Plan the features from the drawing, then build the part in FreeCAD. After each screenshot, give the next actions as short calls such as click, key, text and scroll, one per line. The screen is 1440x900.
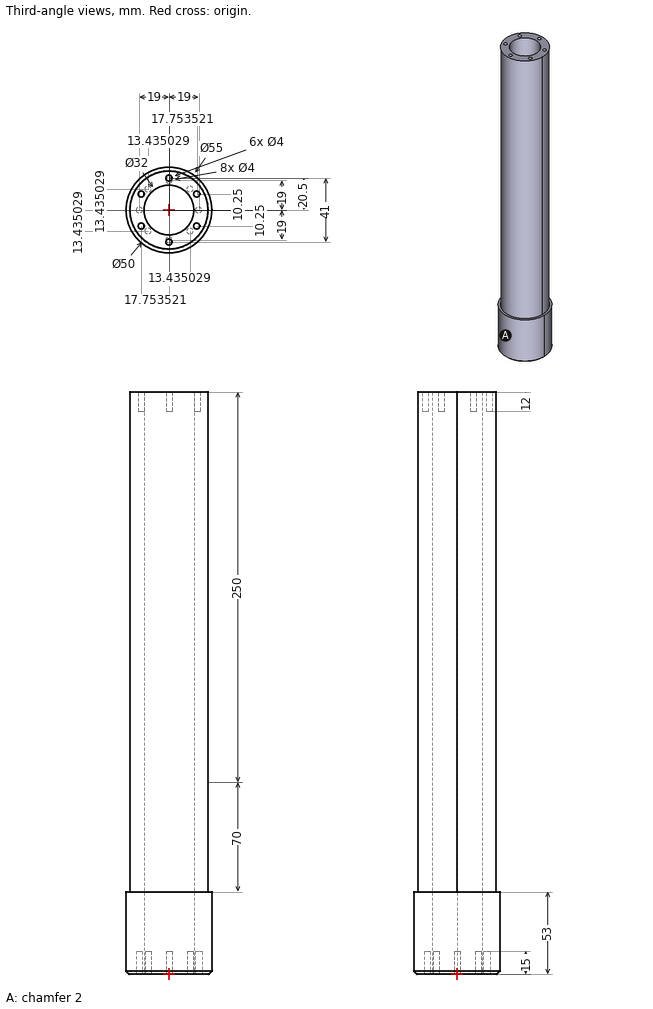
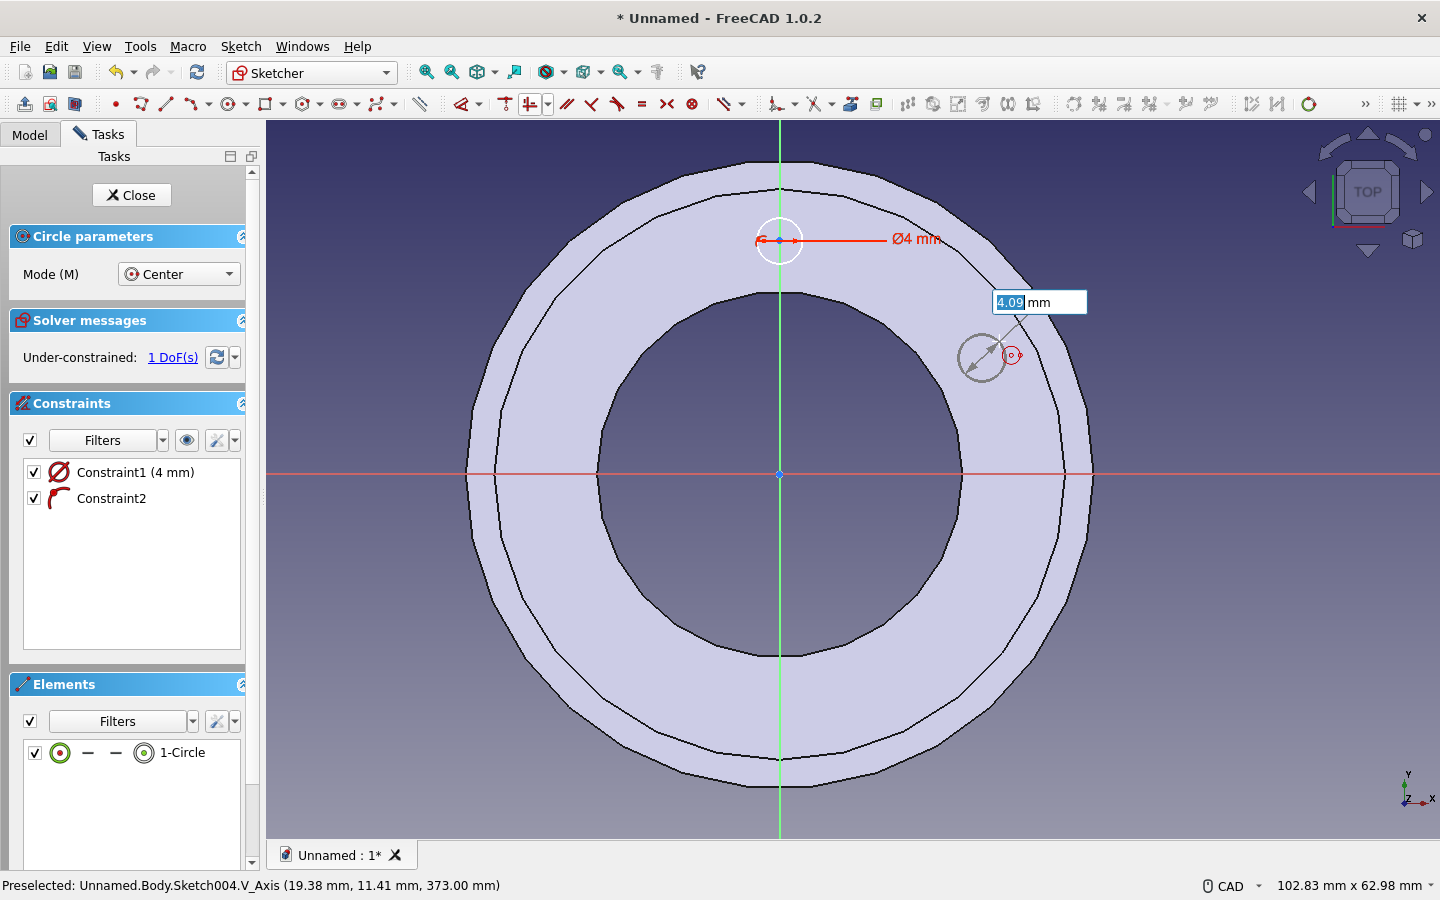
text(4)
key(Return)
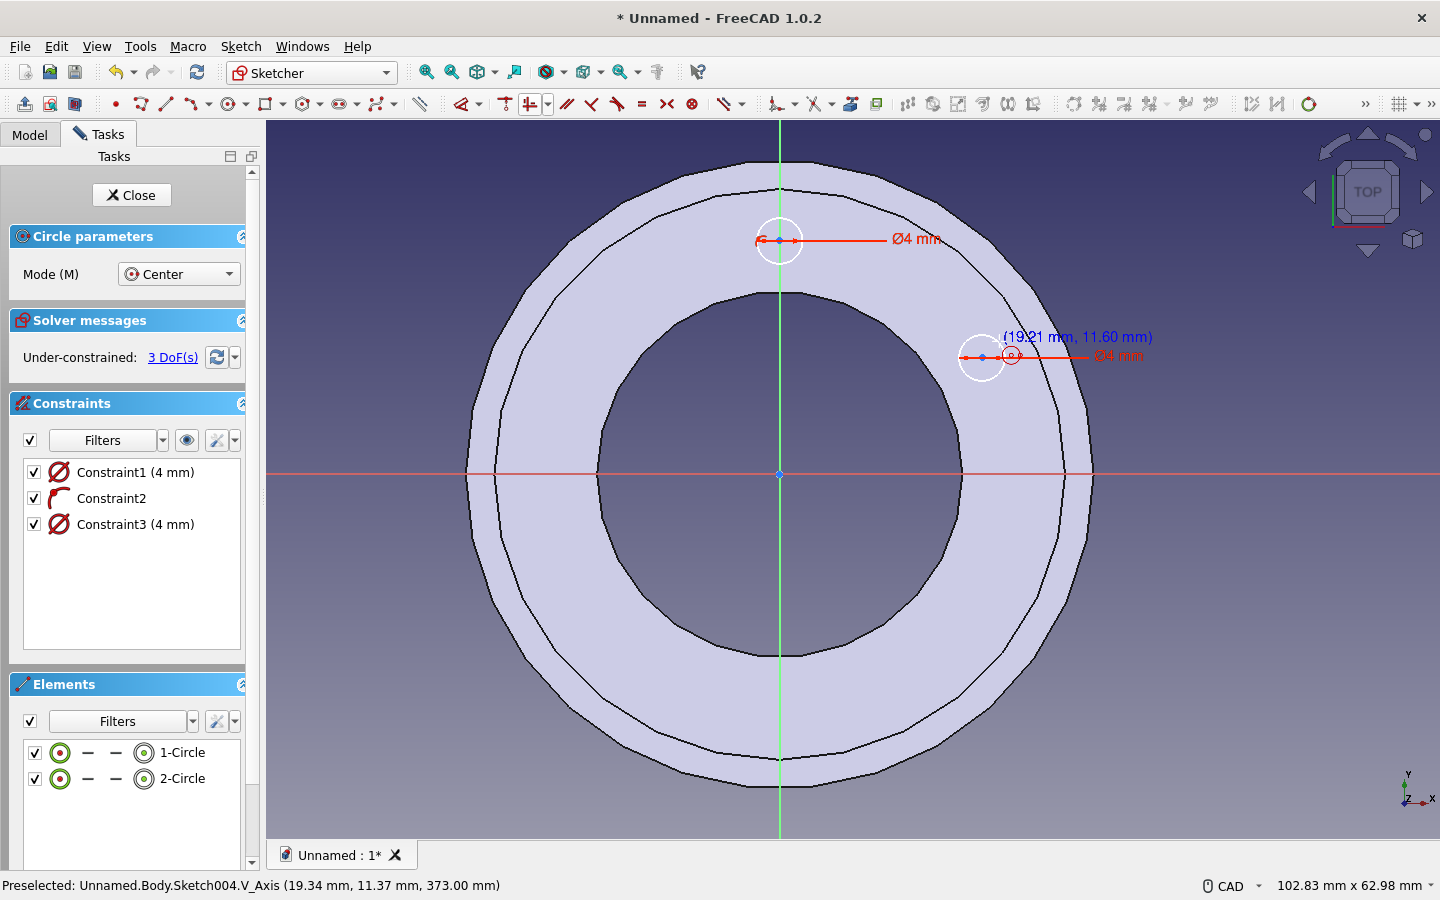
click(982, 591)
move(999, 575)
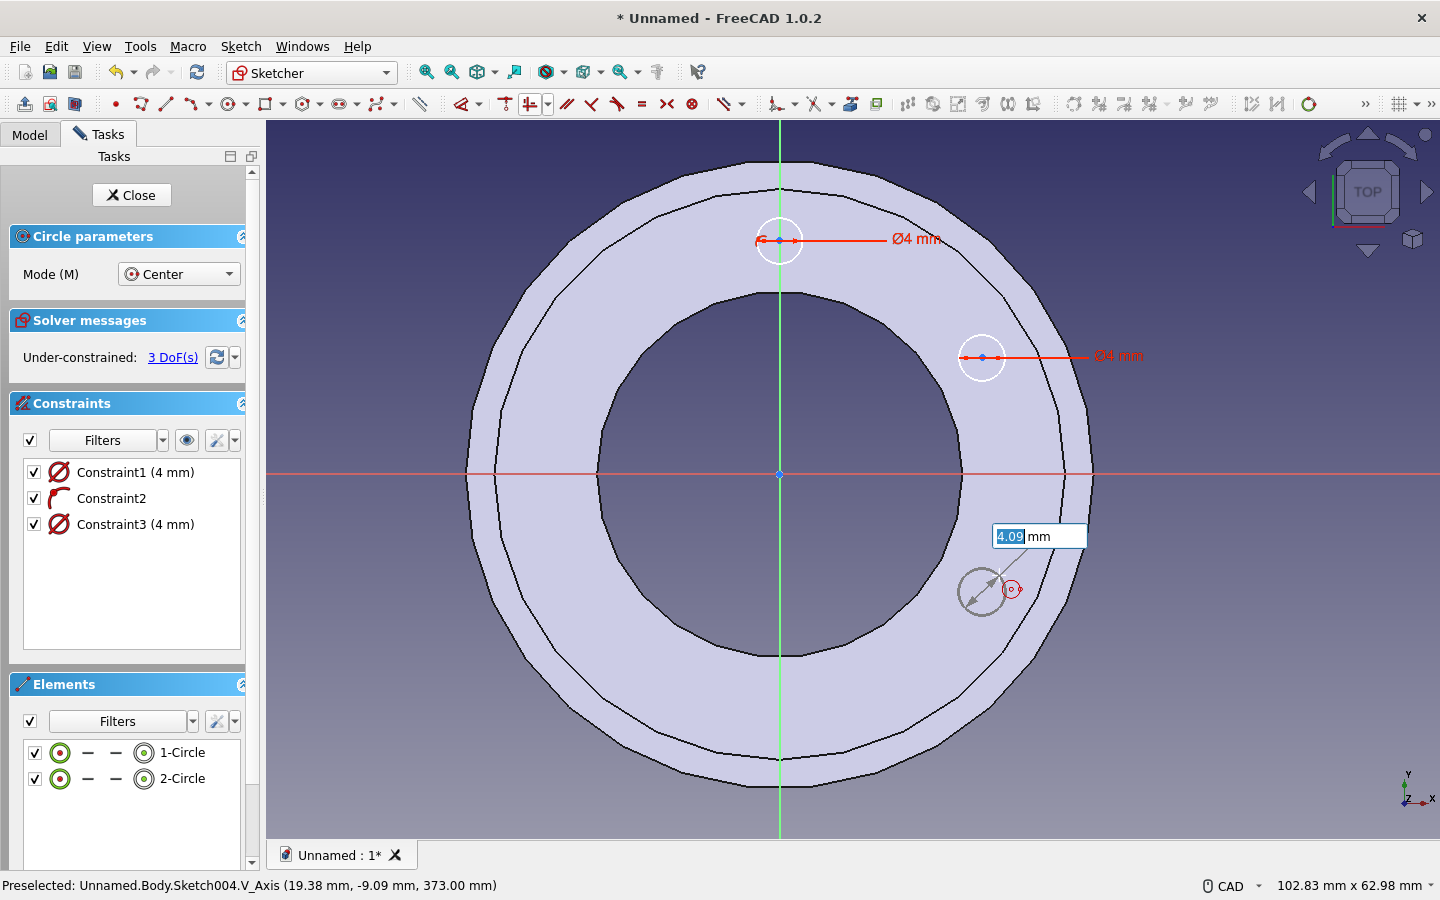
text(4)
key(Return)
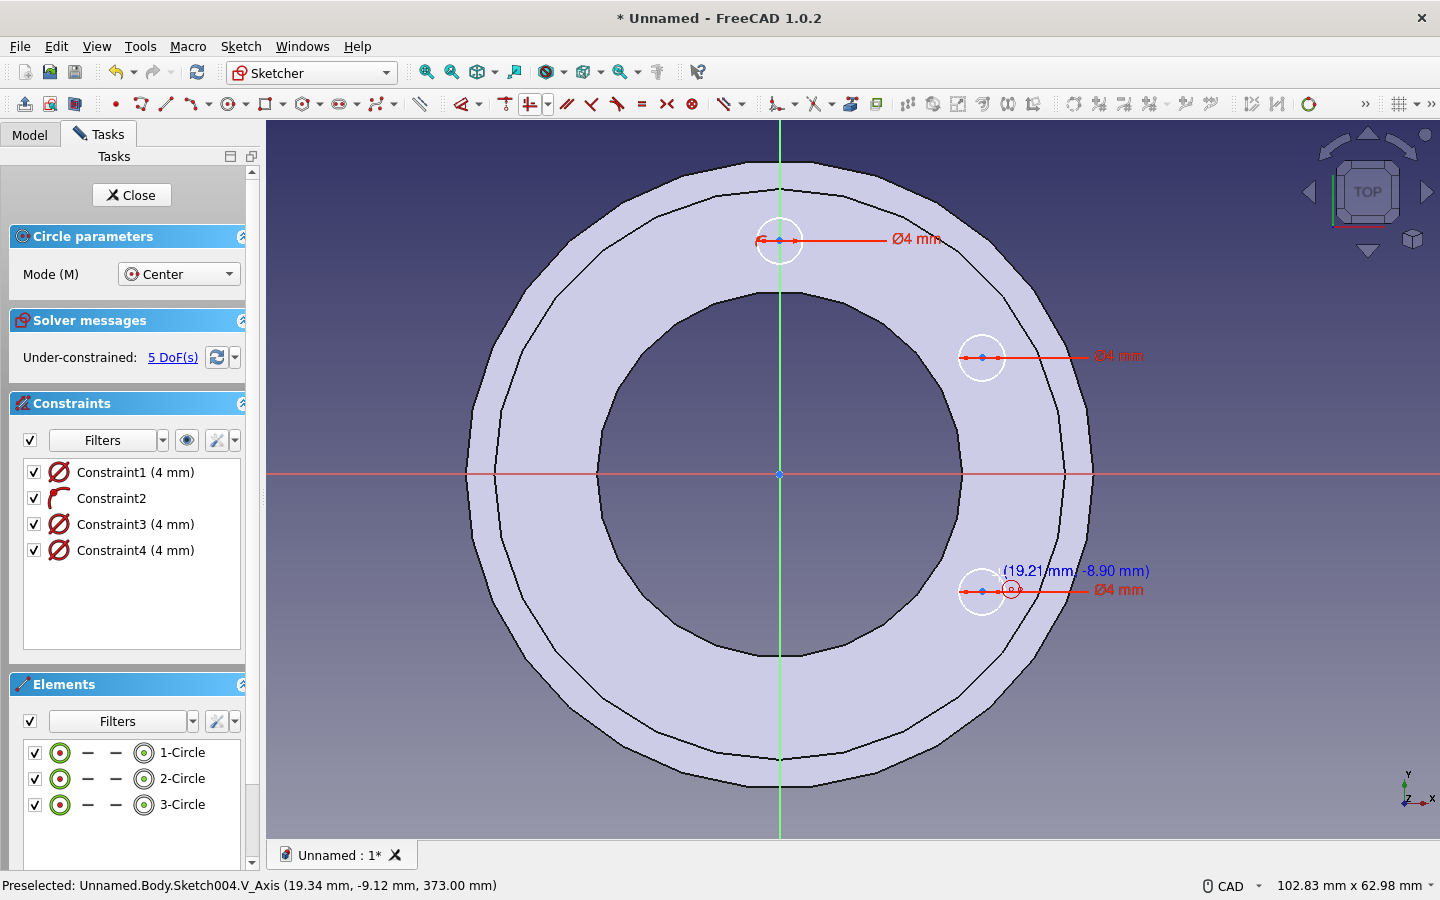
click(780, 708)
move(796, 692)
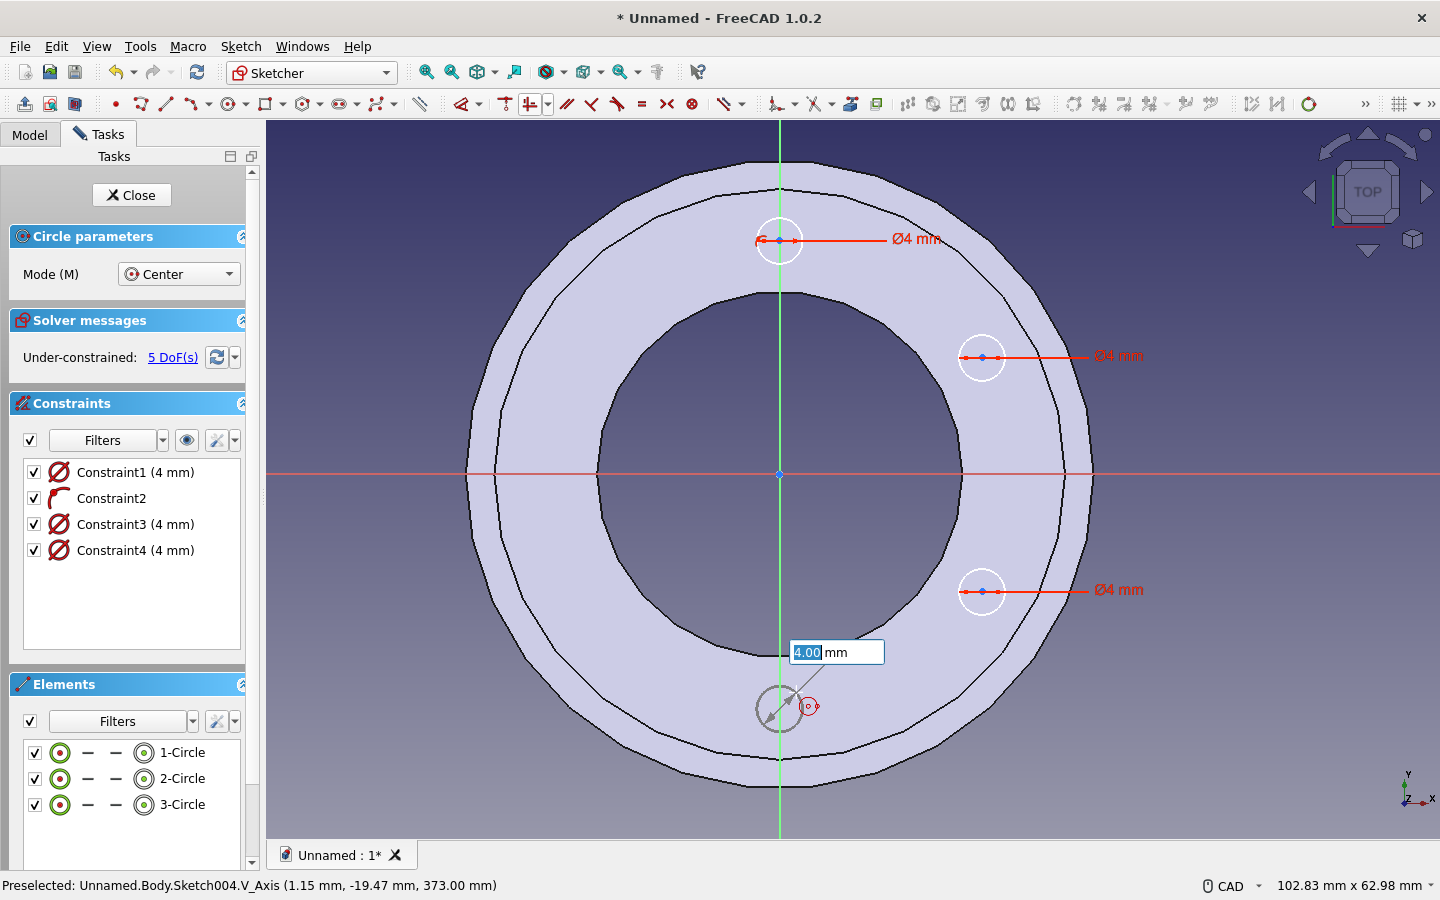
text(4)
key(Return)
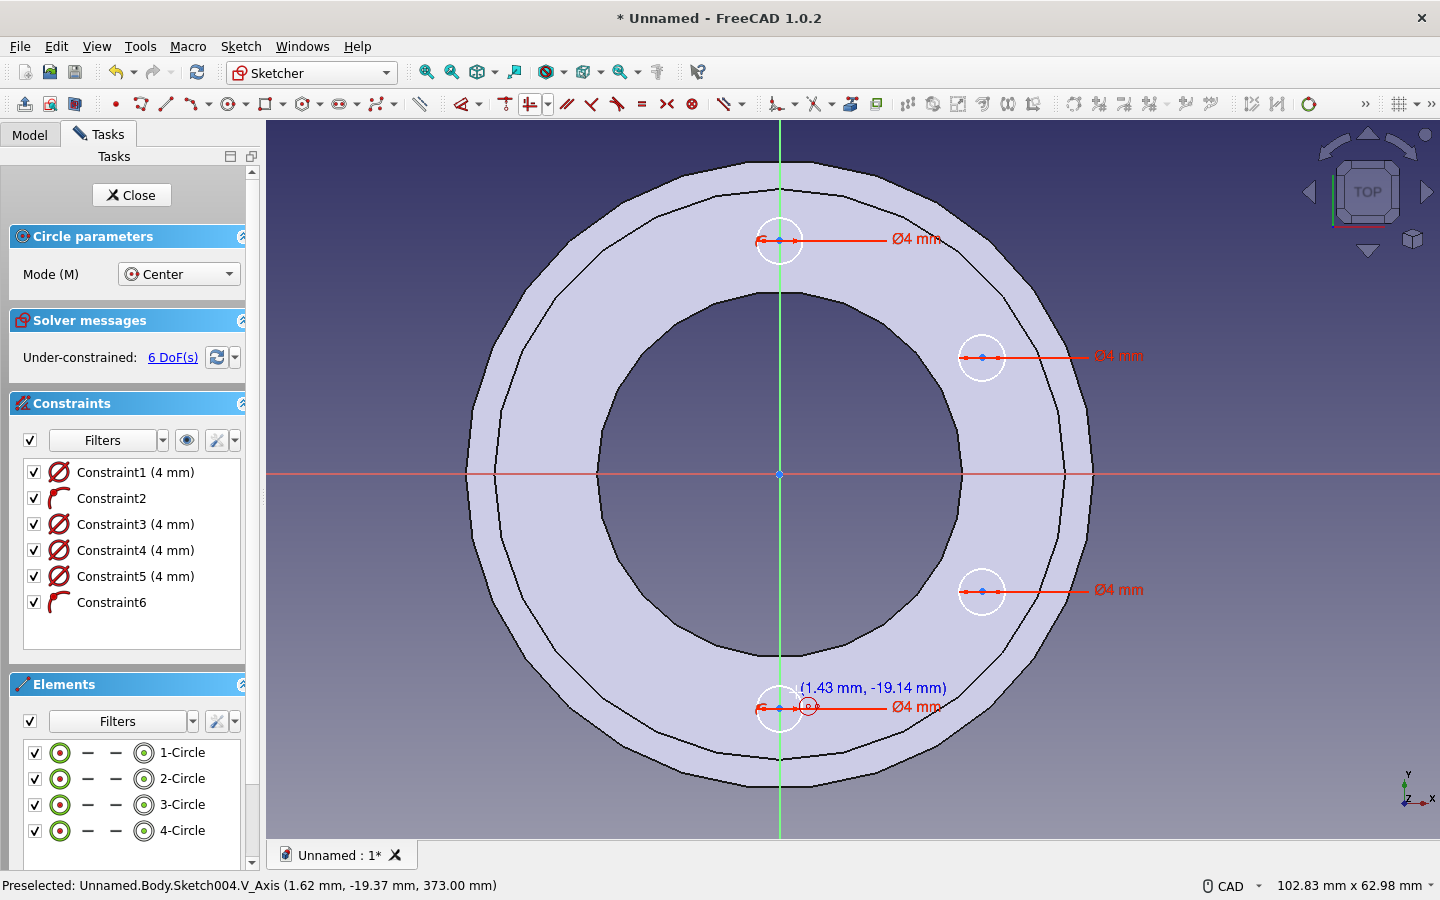
click(577, 591)
move(593, 575)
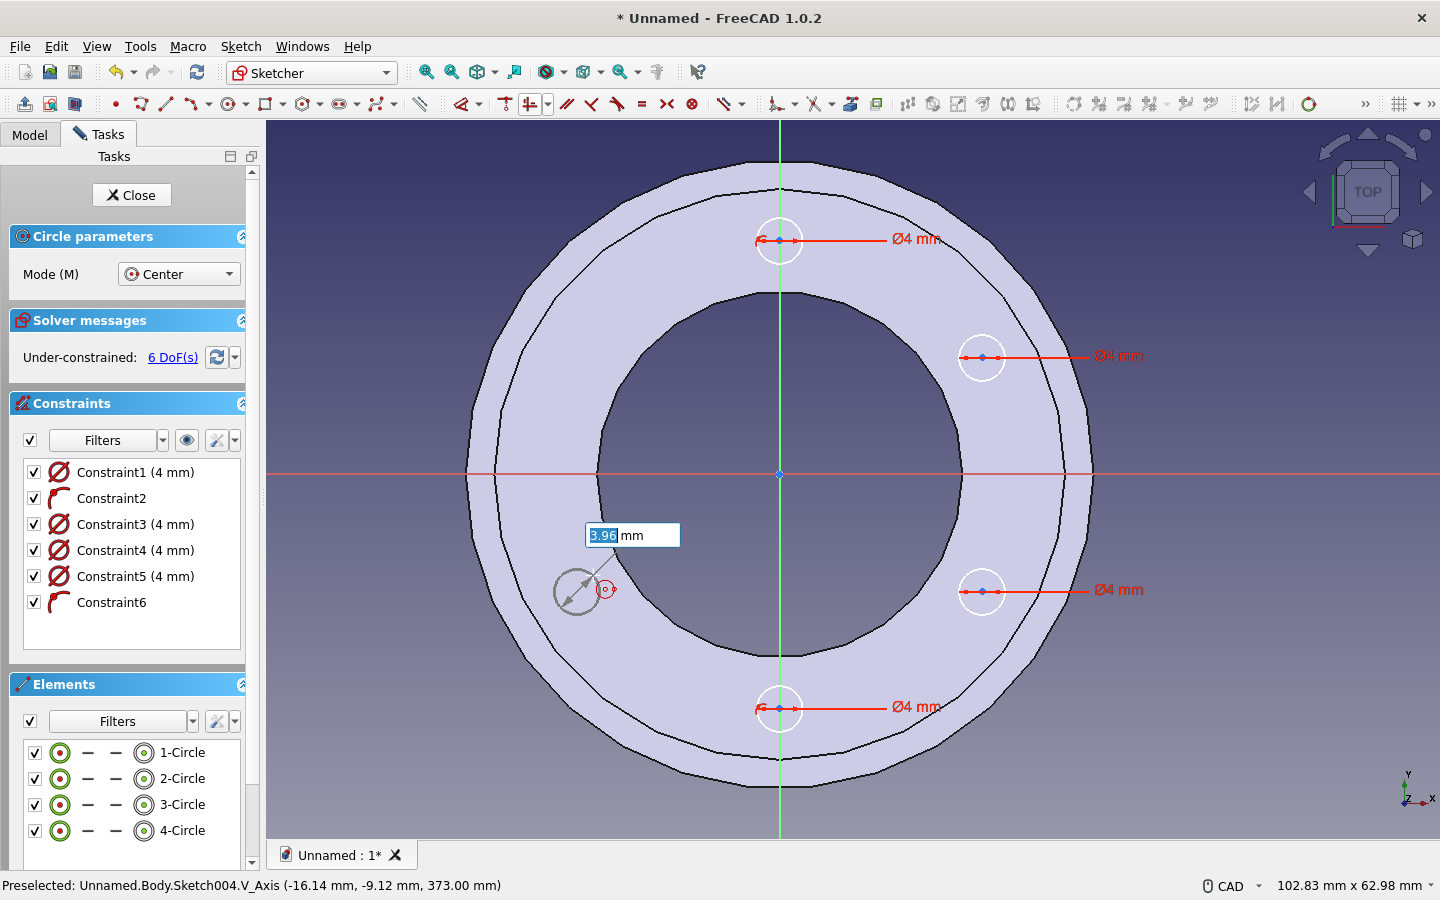
text(4)
key(Return)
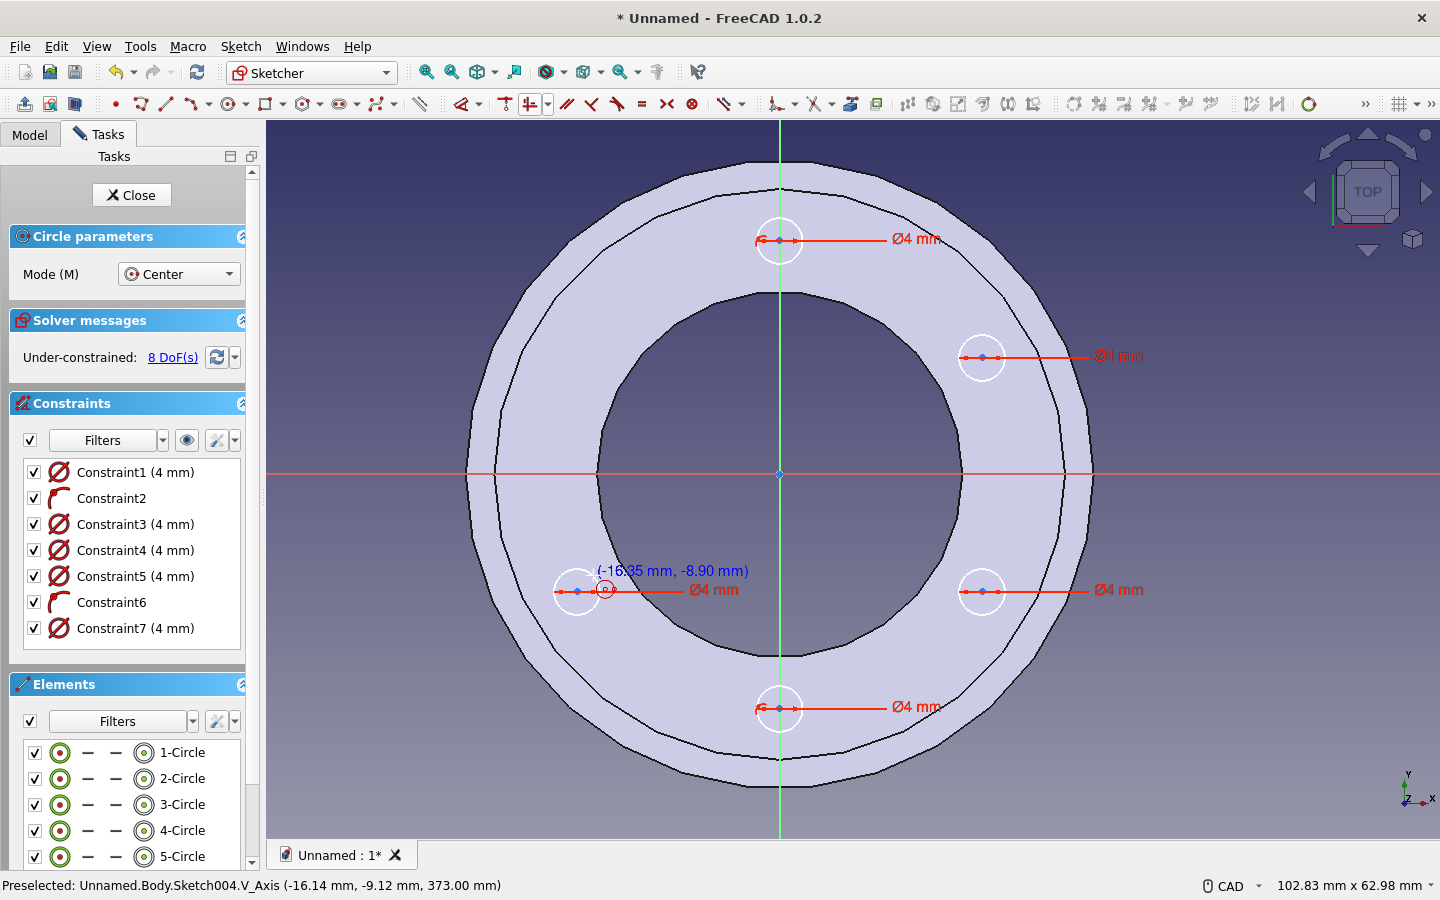
click(577, 357)
move(593, 341)